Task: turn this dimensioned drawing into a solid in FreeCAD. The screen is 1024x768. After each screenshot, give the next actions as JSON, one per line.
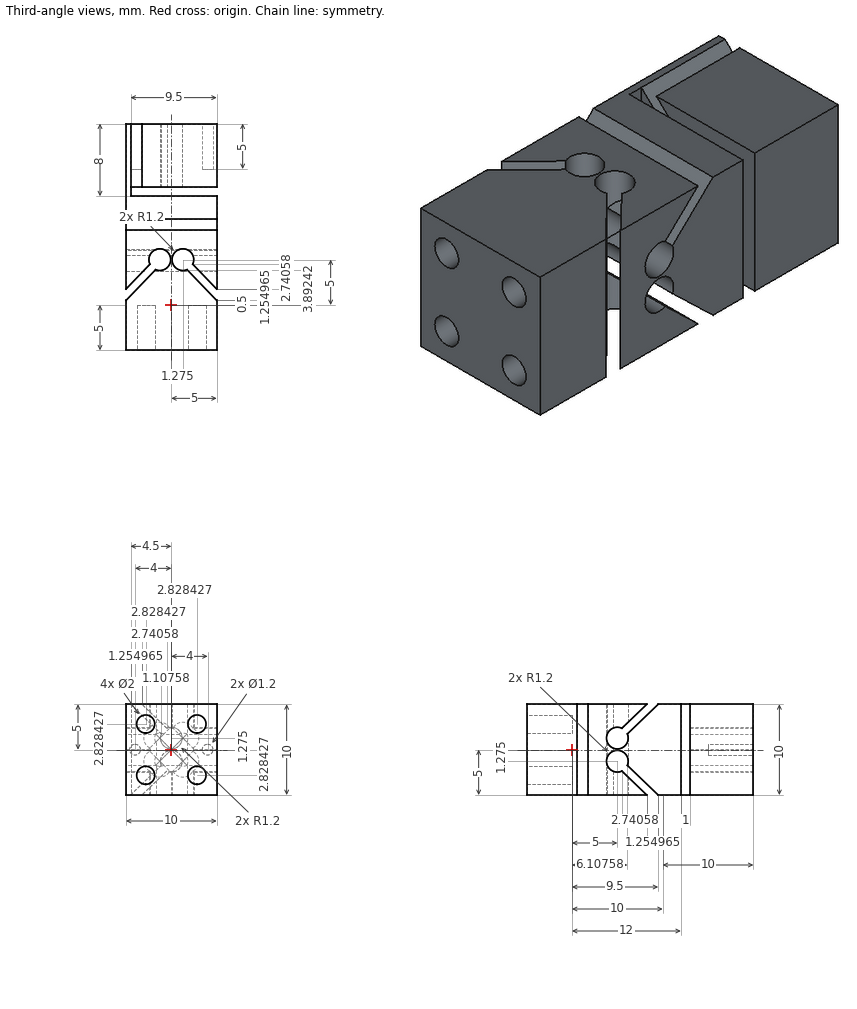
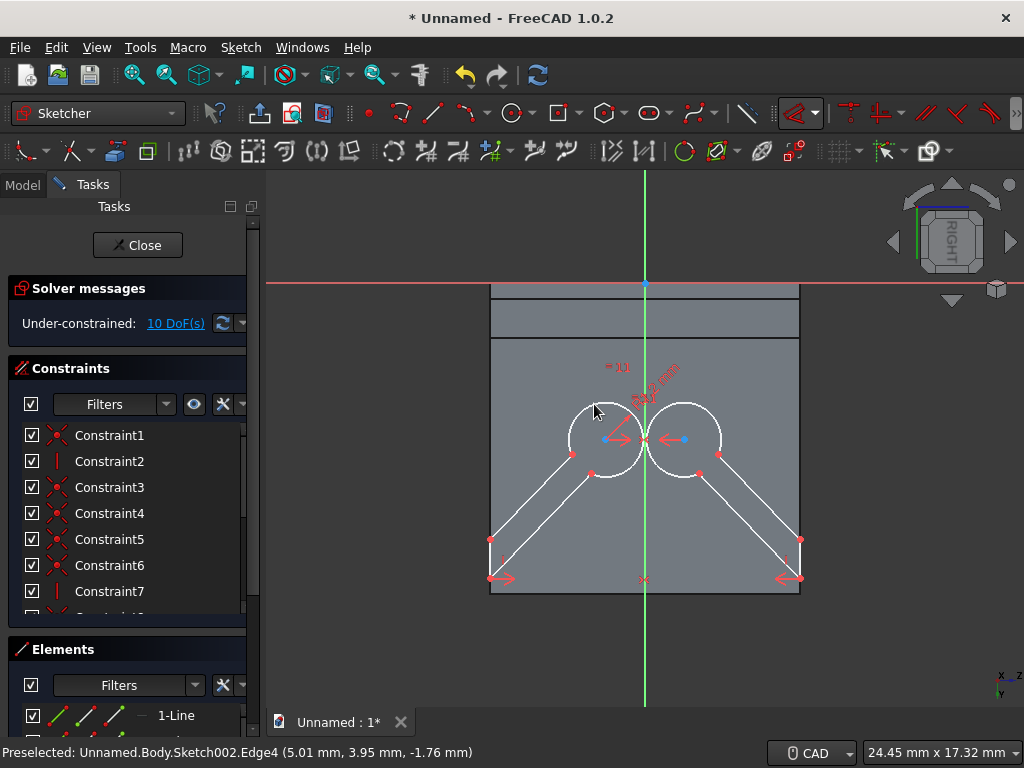
{"action": "left_click", "coordinate": [490, 540]}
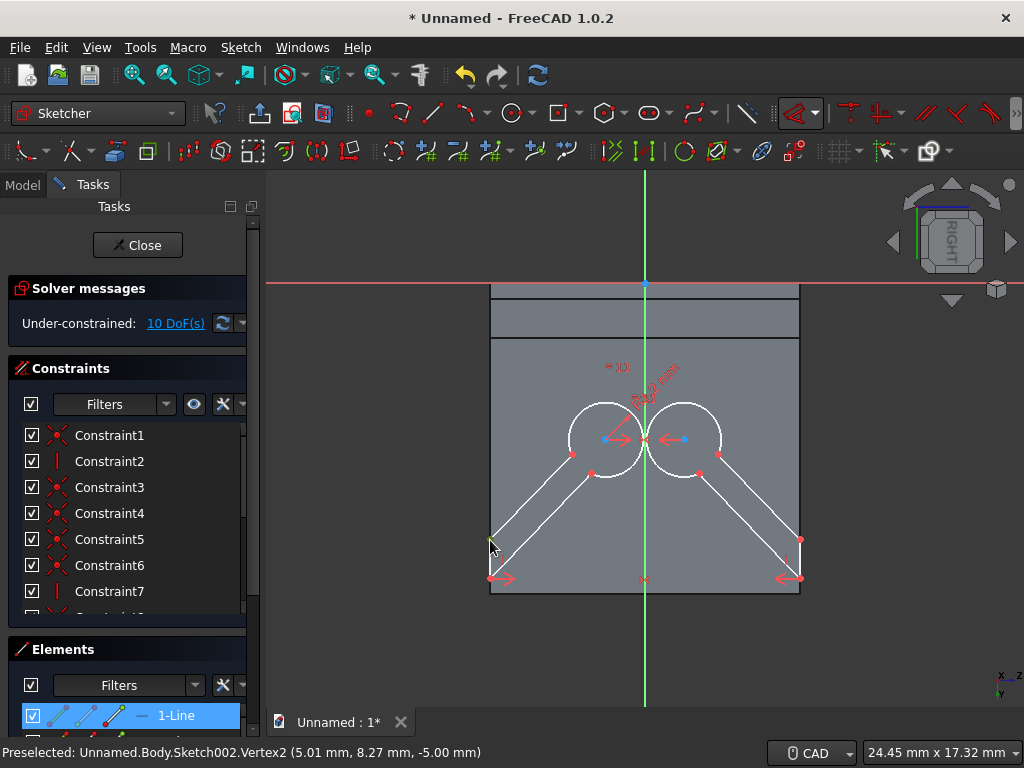
{"action": "key", "text": "l"}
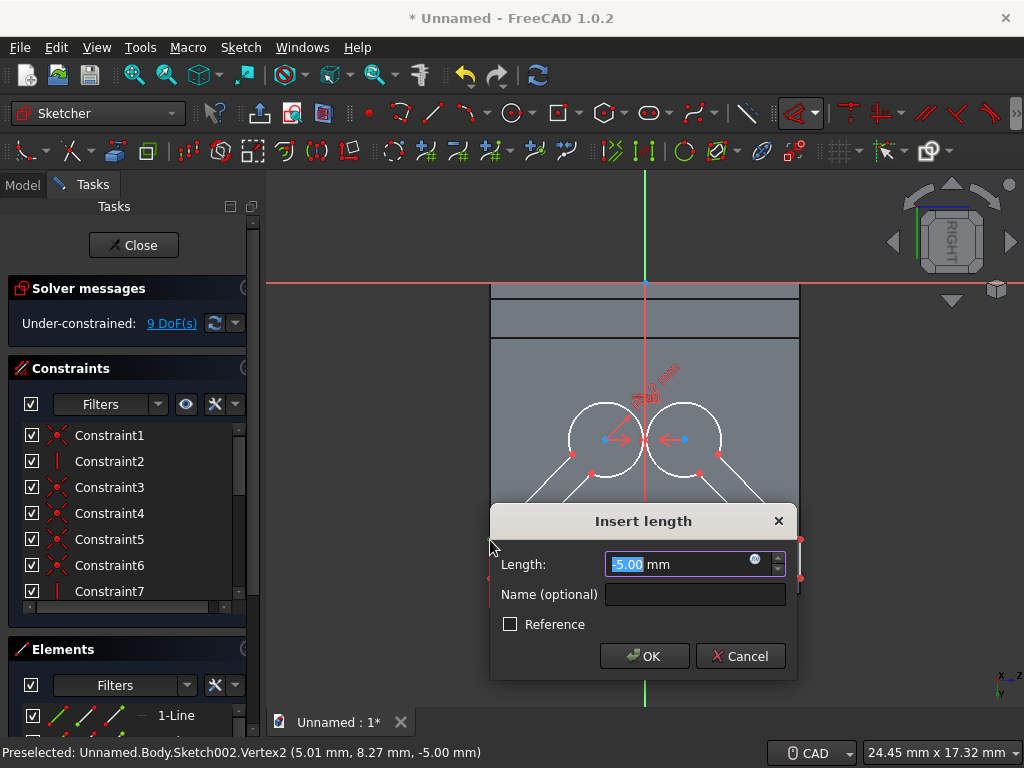
{"action": "type", "text": "-5"}
{"action": "key", "text": "Return"}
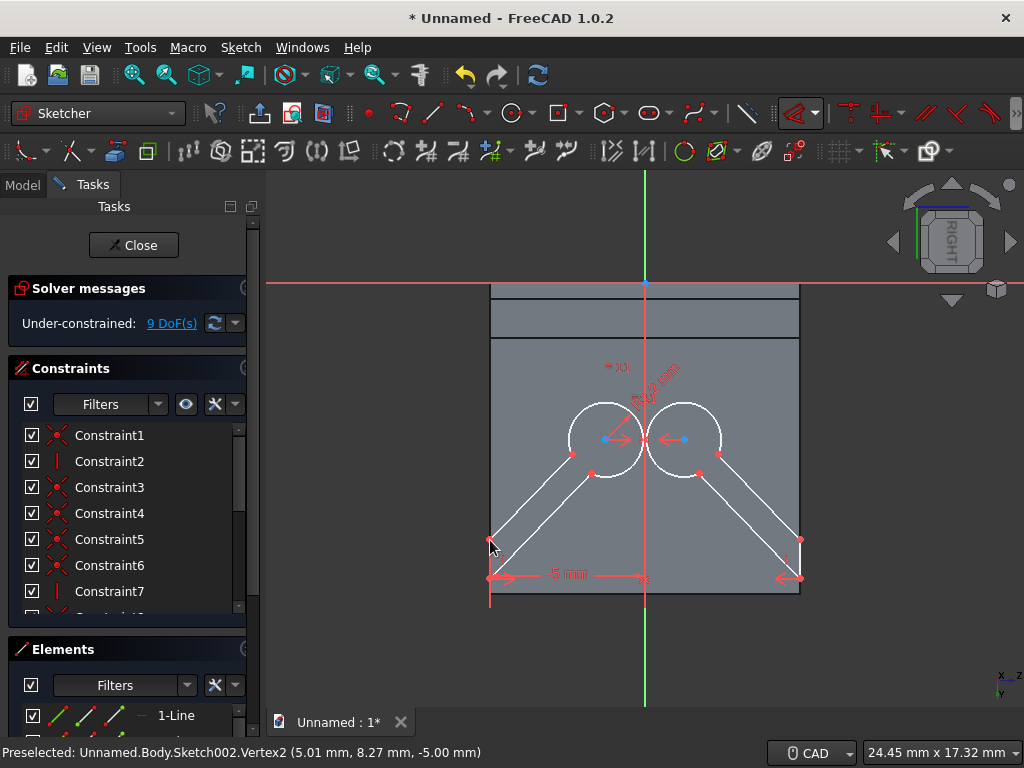
{"action": "left_click", "coordinate": [606, 440]}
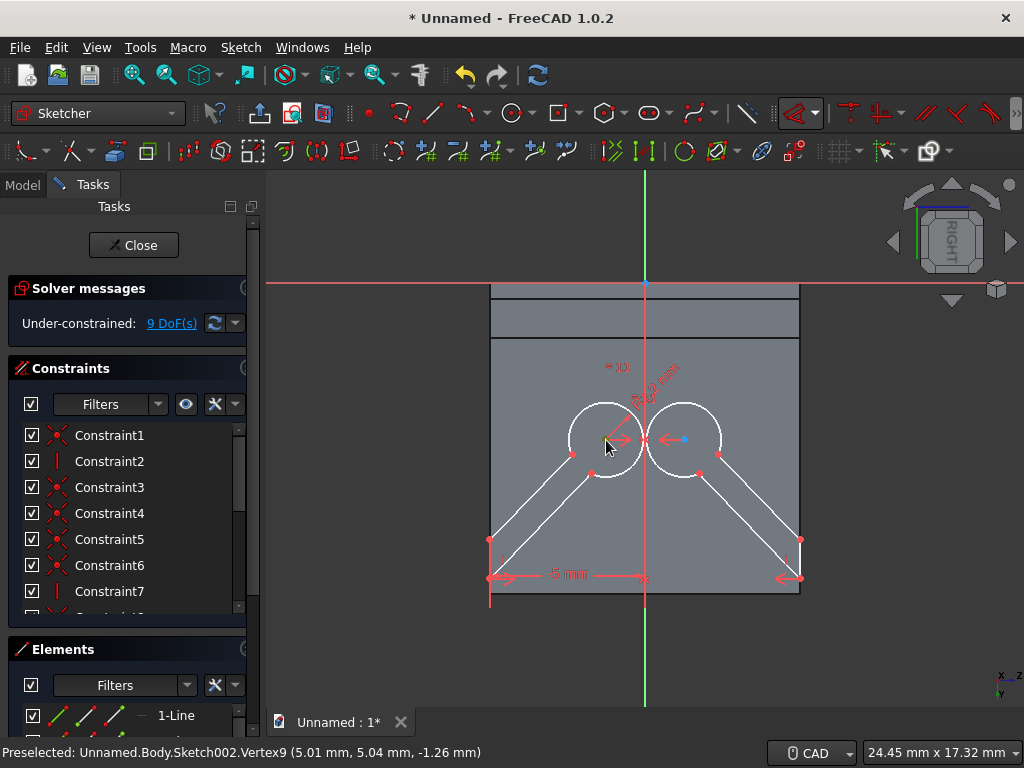
{"action": "key", "text": "i"}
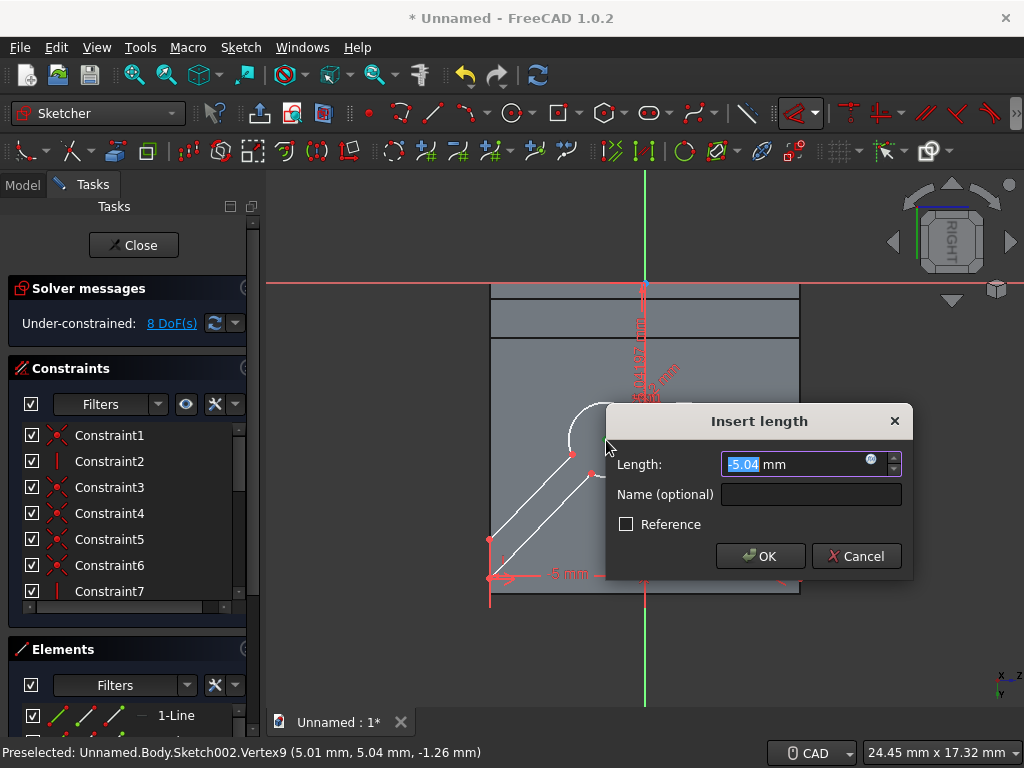
{"action": "type", "text": "-5"}
{"action": "key", "text": "Return"}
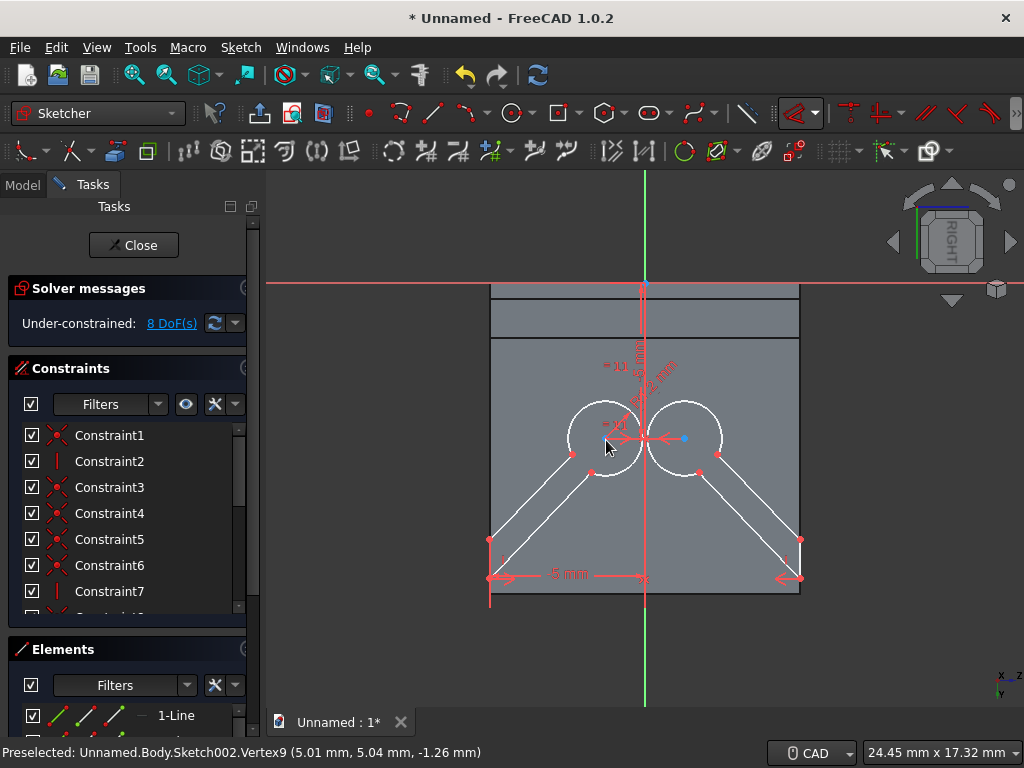
{"action": "left_click", "coordinate": [490, 579]}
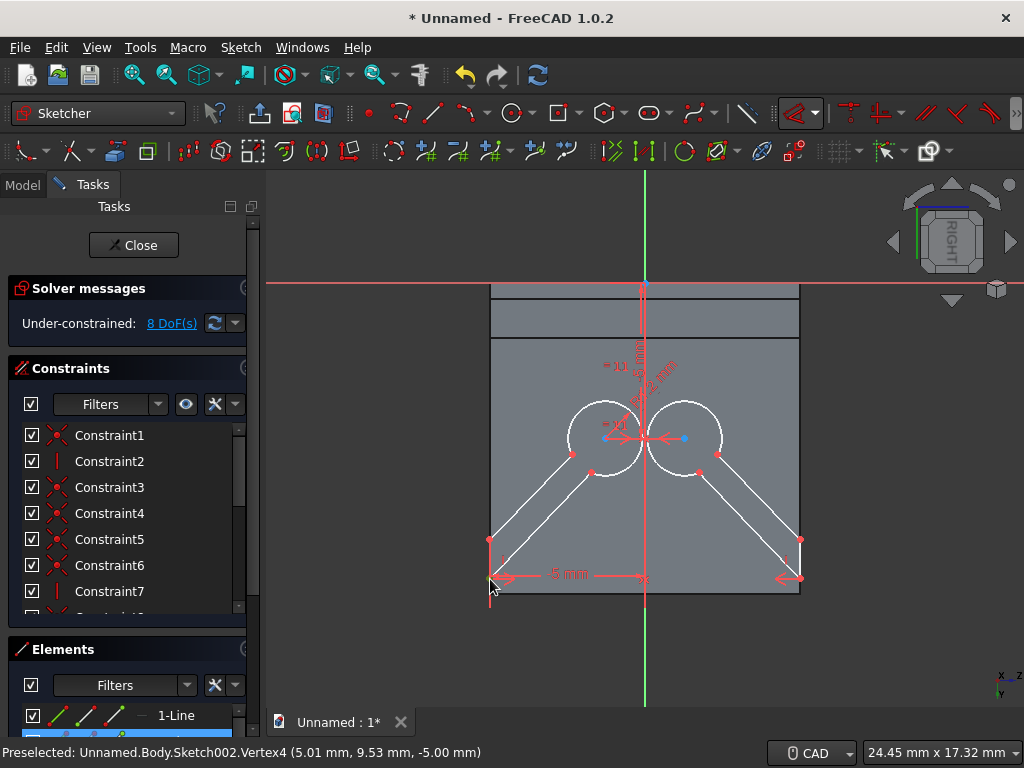
{"action": "key", "text": "i"}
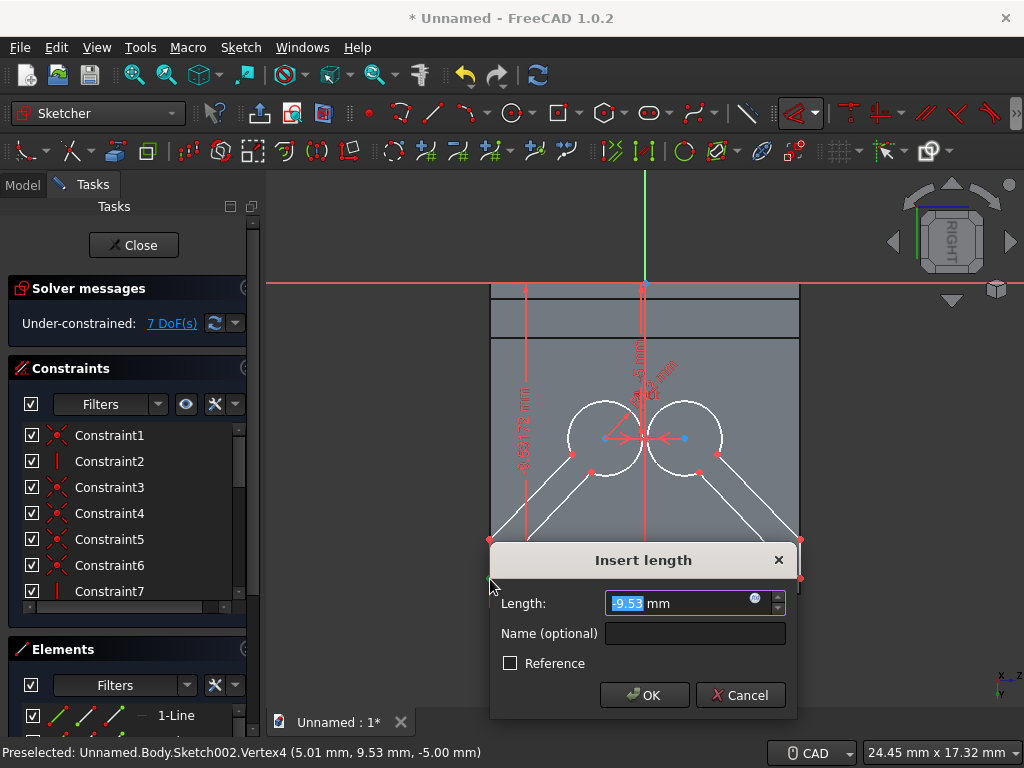
{"action": "type", "text": "-9.5"}
{"action": "key", "text": "Return"}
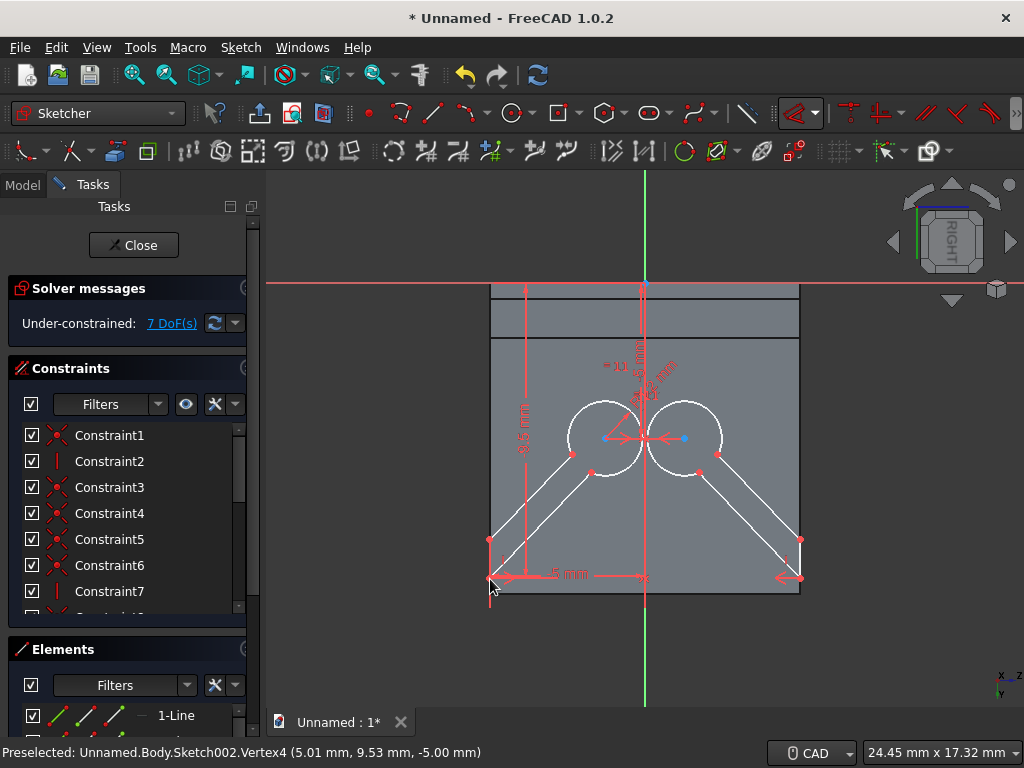
{"action": "left_click", "coordinate": [605, 438]}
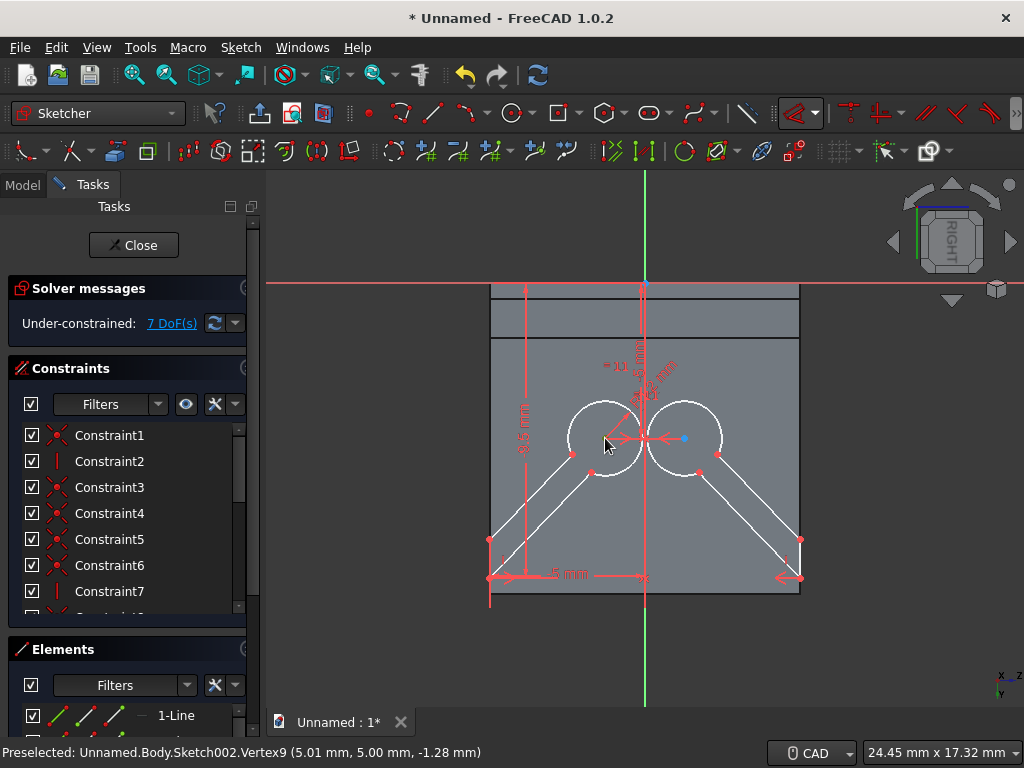
{"action": "key", "text": "l"}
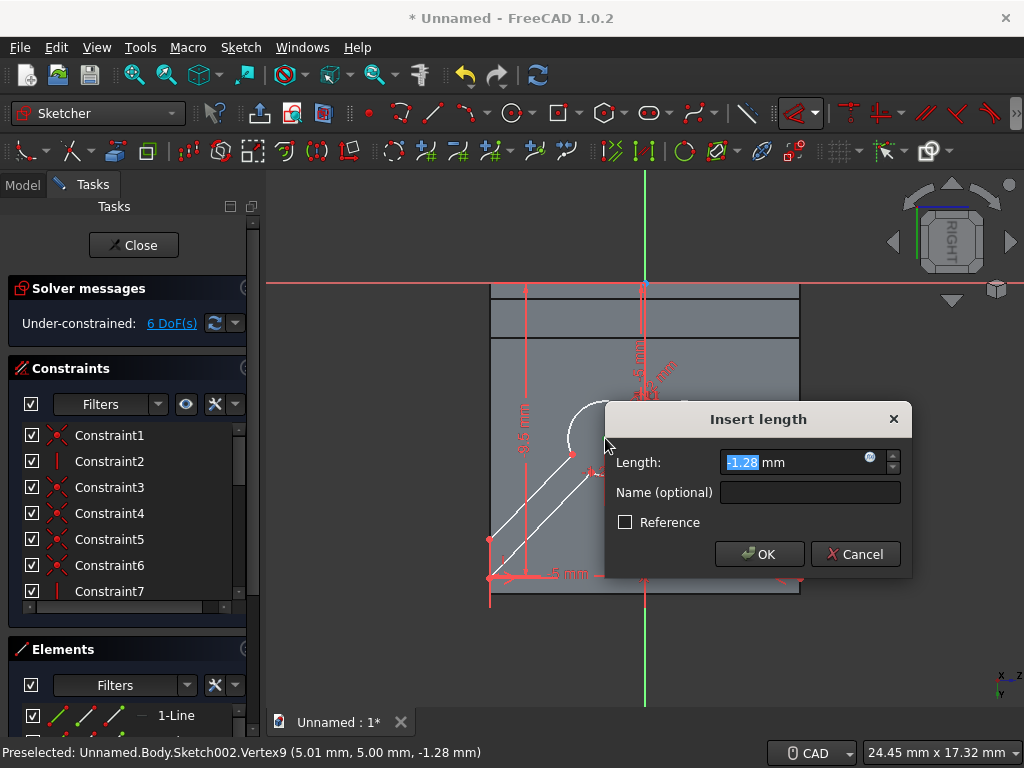
{"action": "type", "text": "-1.275"}
{"action": "key", "text": "Return"}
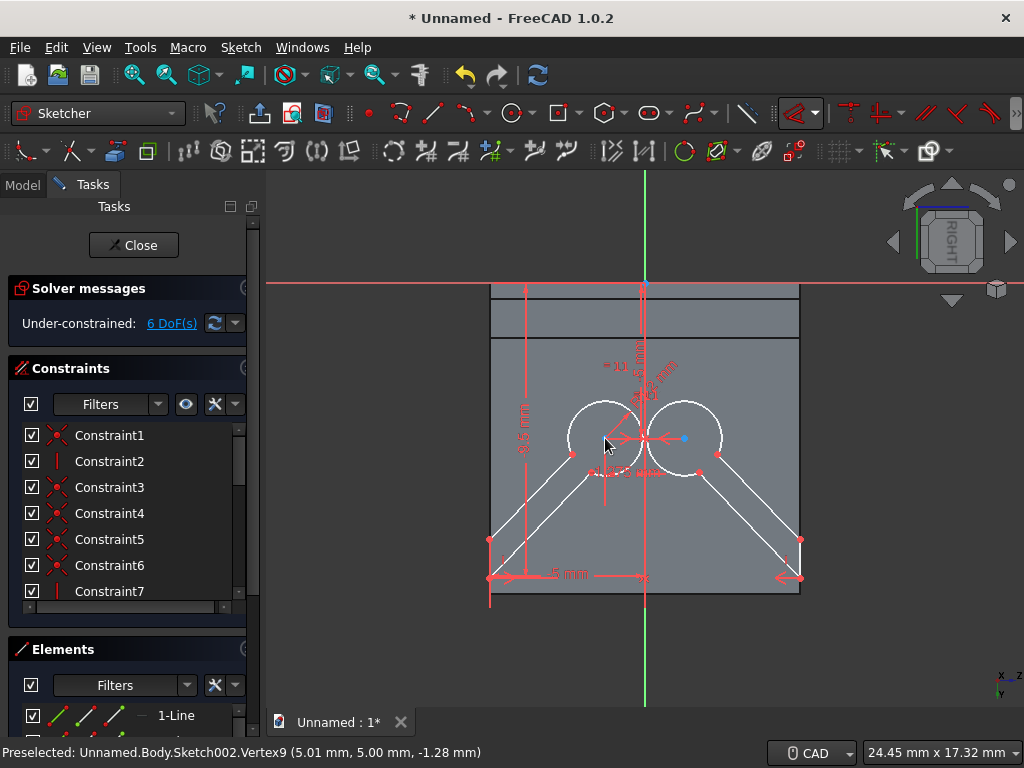
{"action": "left_click", "coordinate": [490, 551]}